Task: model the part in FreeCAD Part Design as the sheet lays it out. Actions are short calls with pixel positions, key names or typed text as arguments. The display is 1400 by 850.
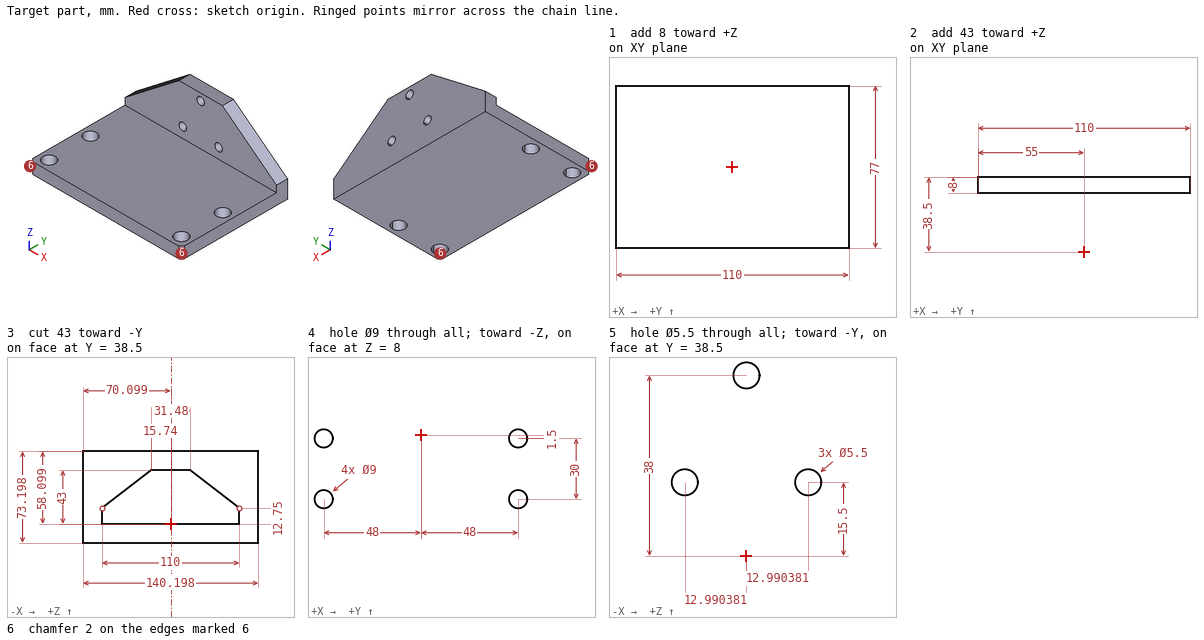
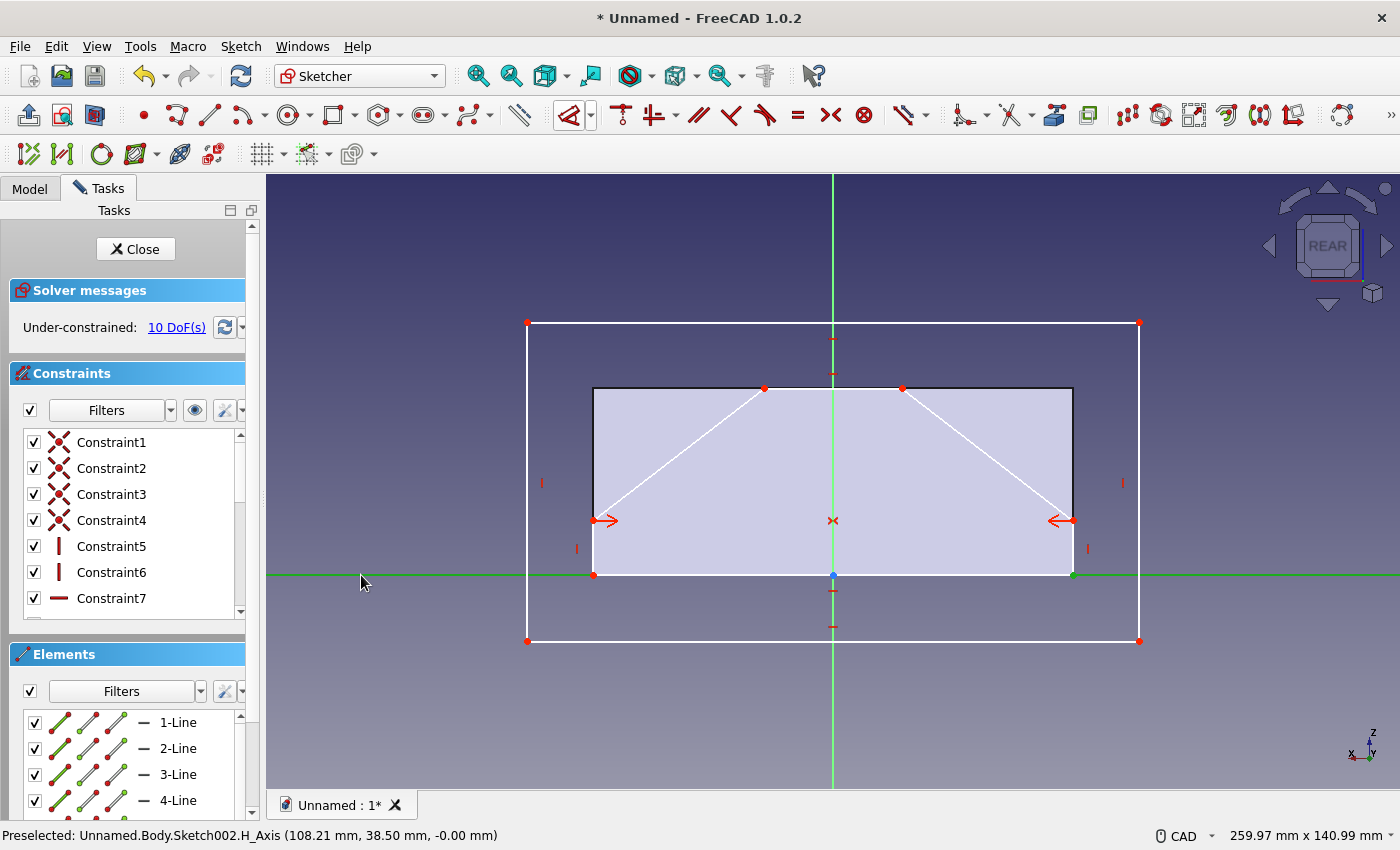
click(621, 116)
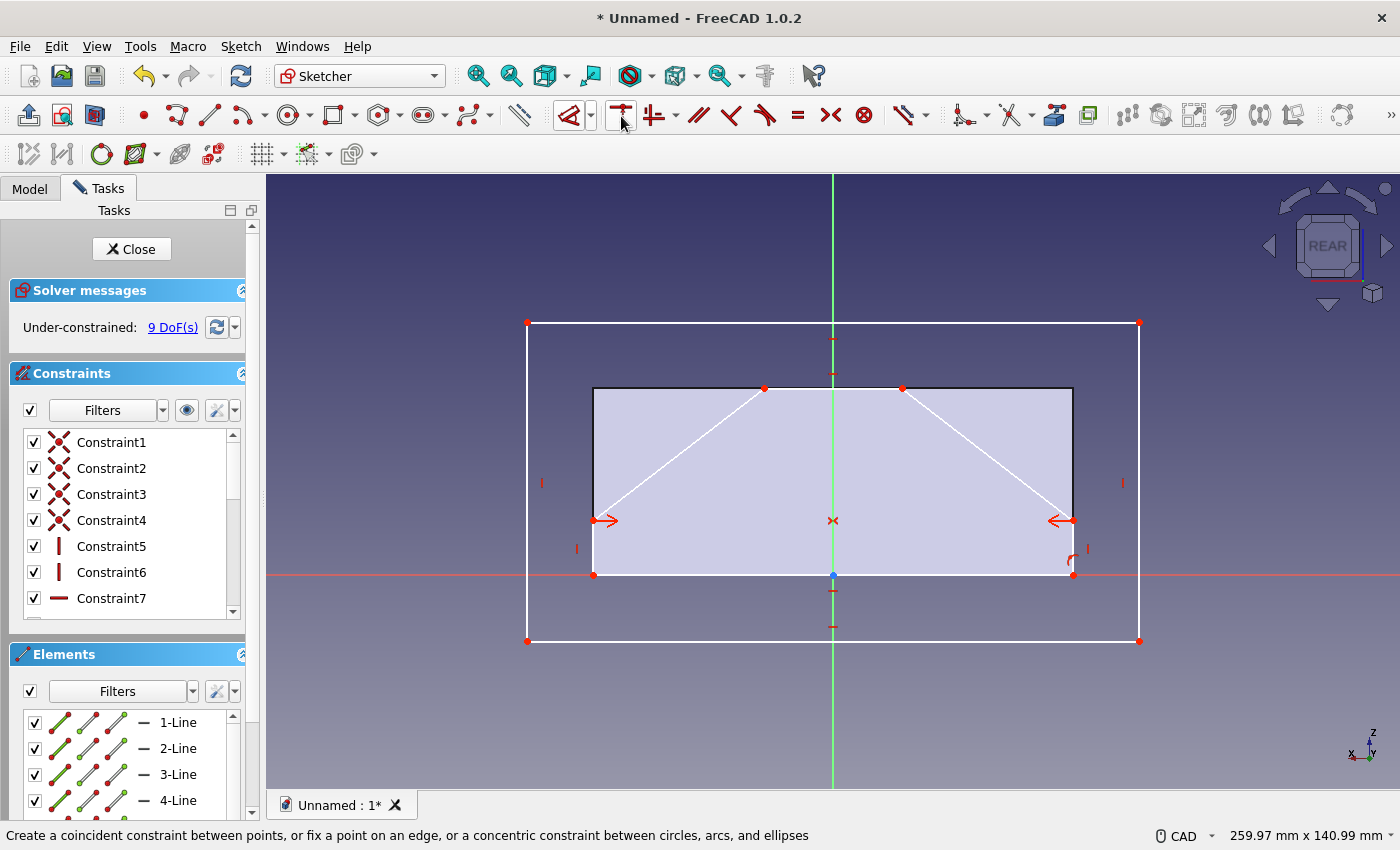
click(929, 575)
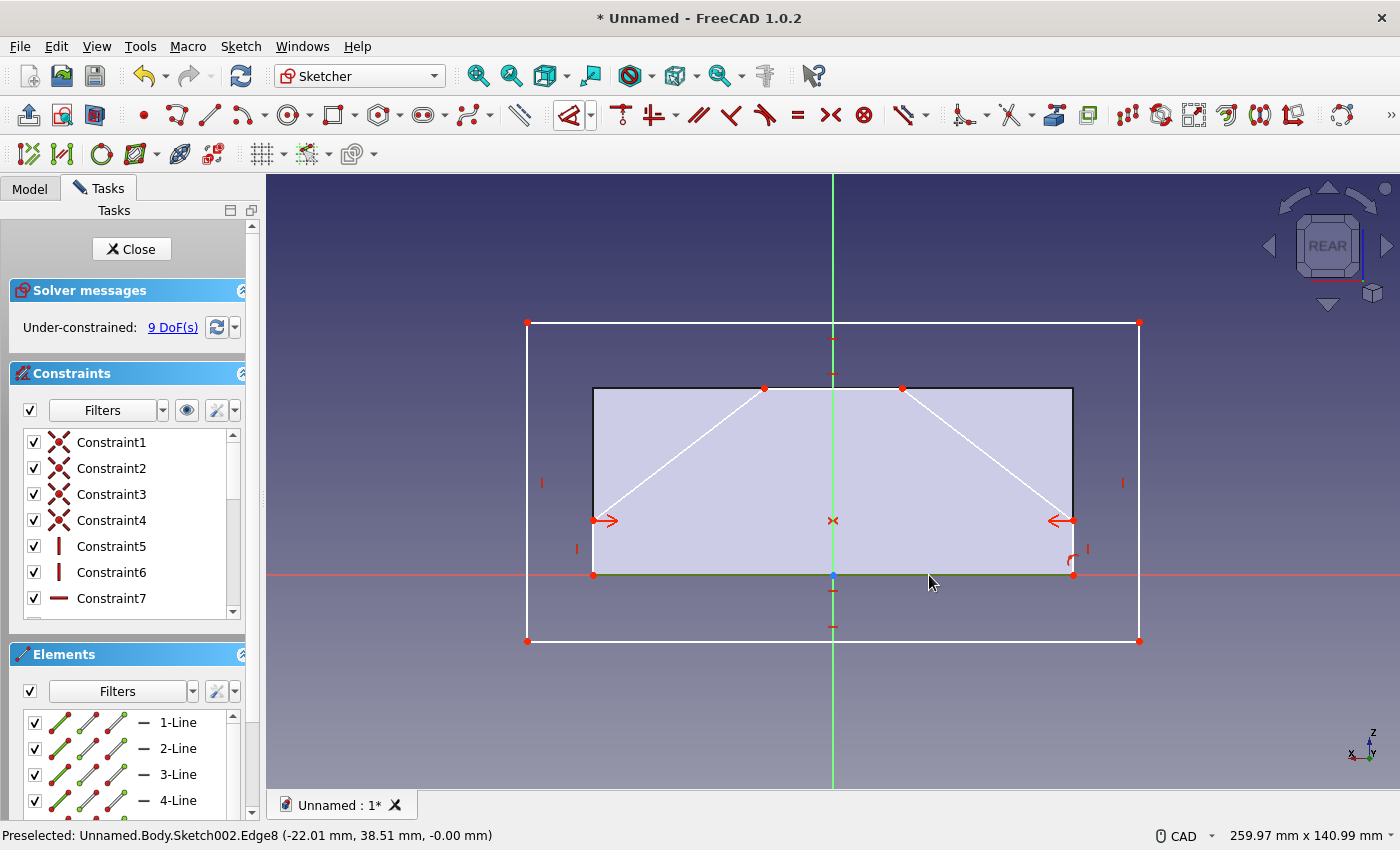
key(l)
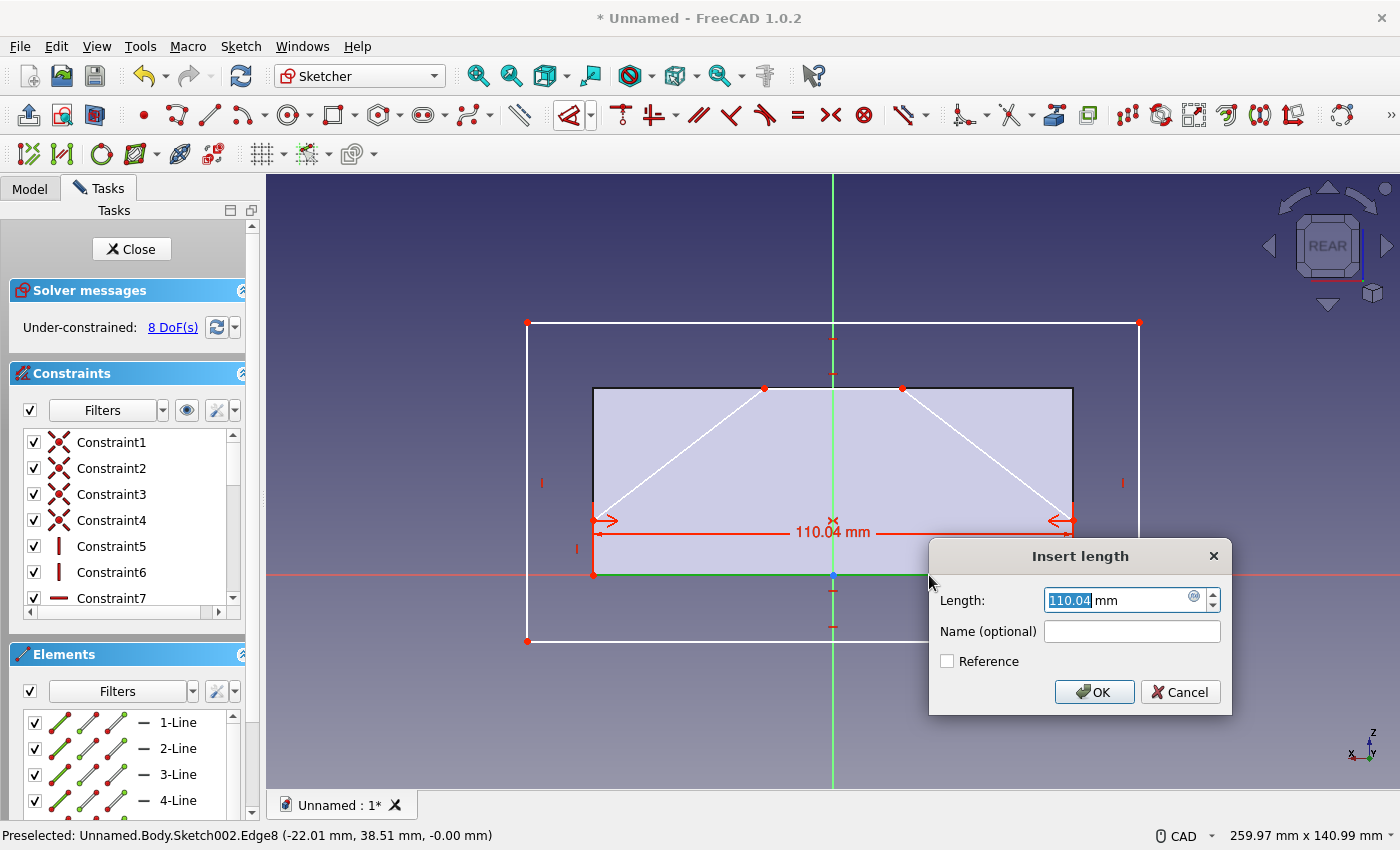
text(110)
key(Return)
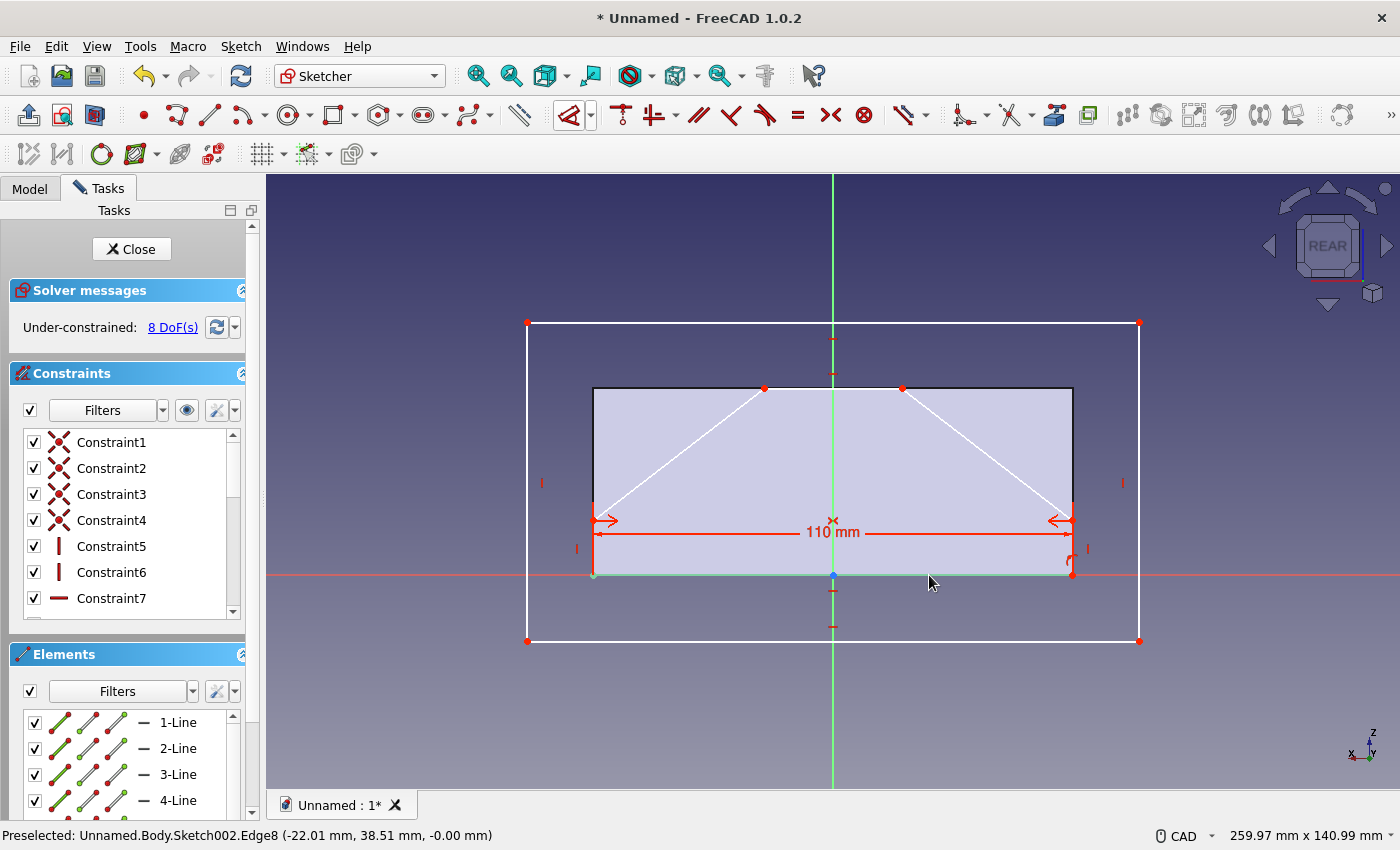
click(764, 389)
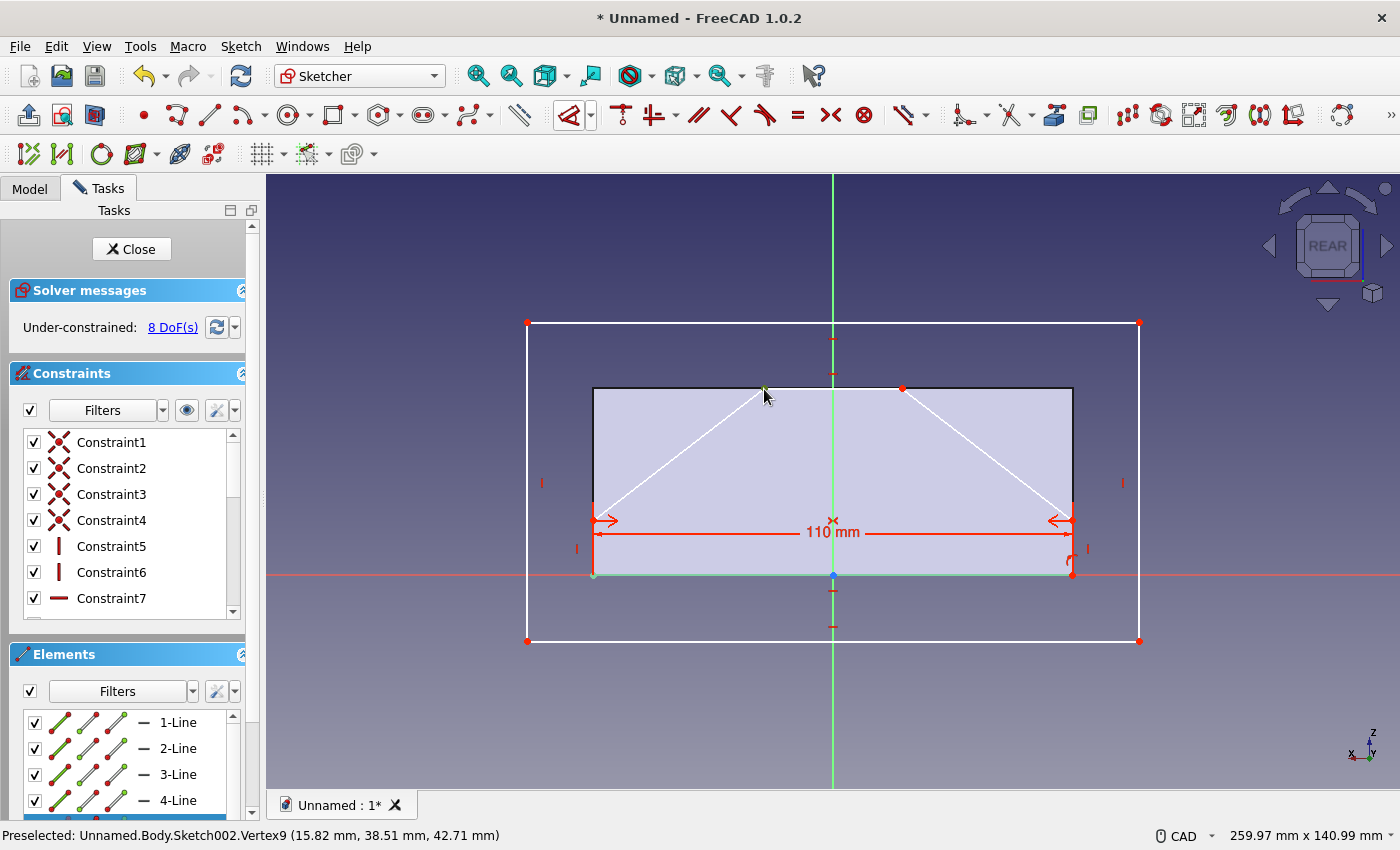
key(i)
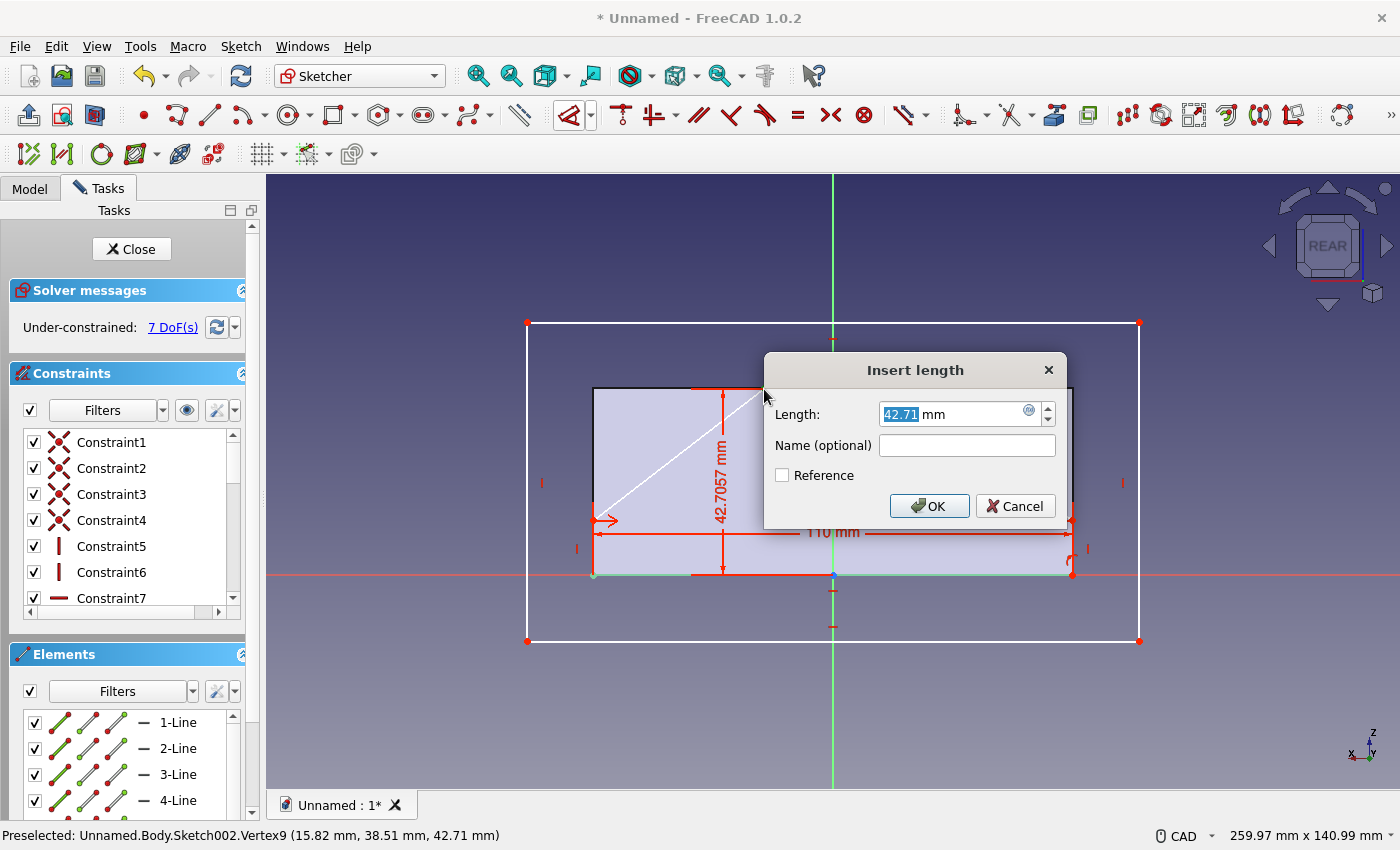
text(43)
key(Return)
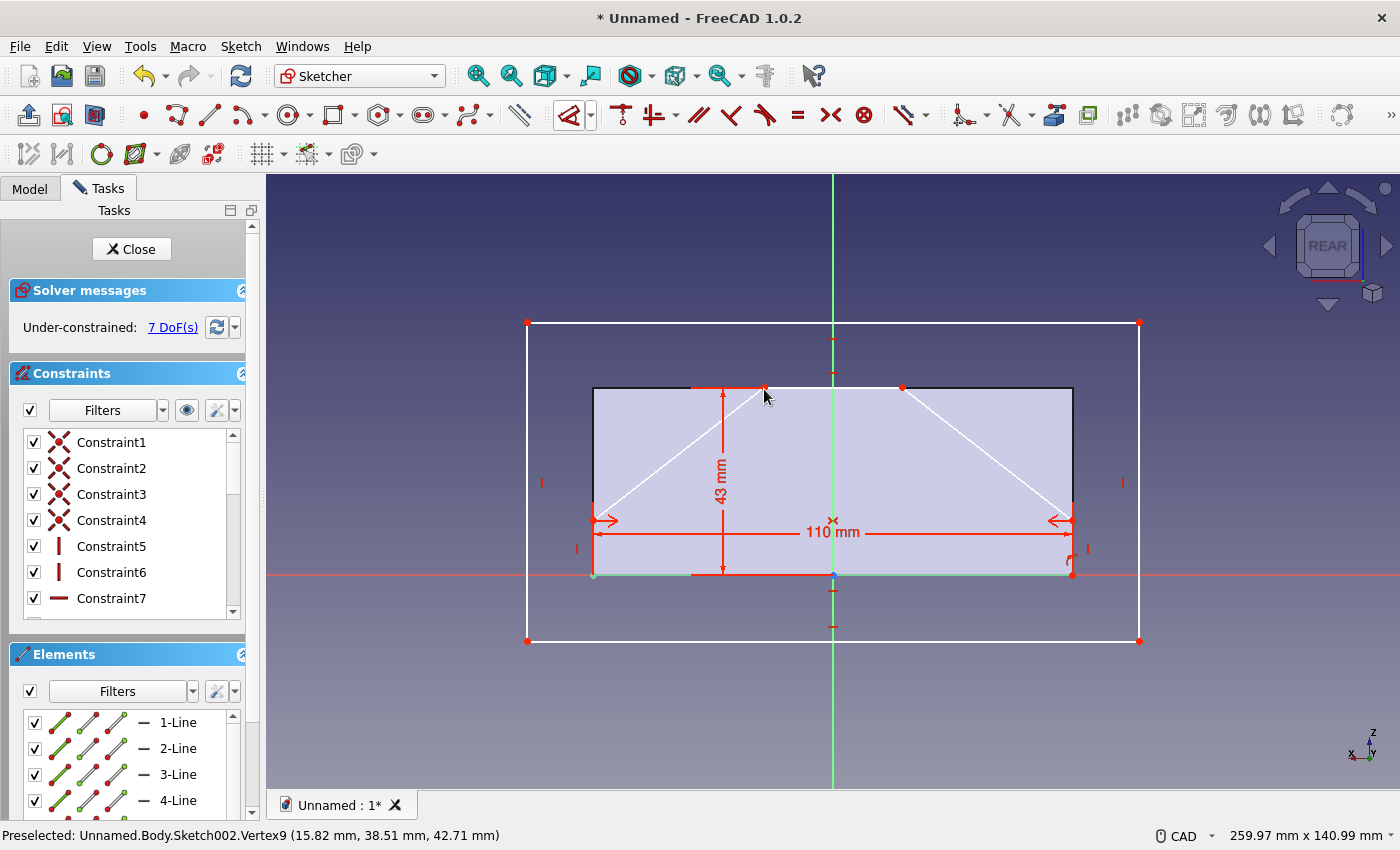
click(805, 388)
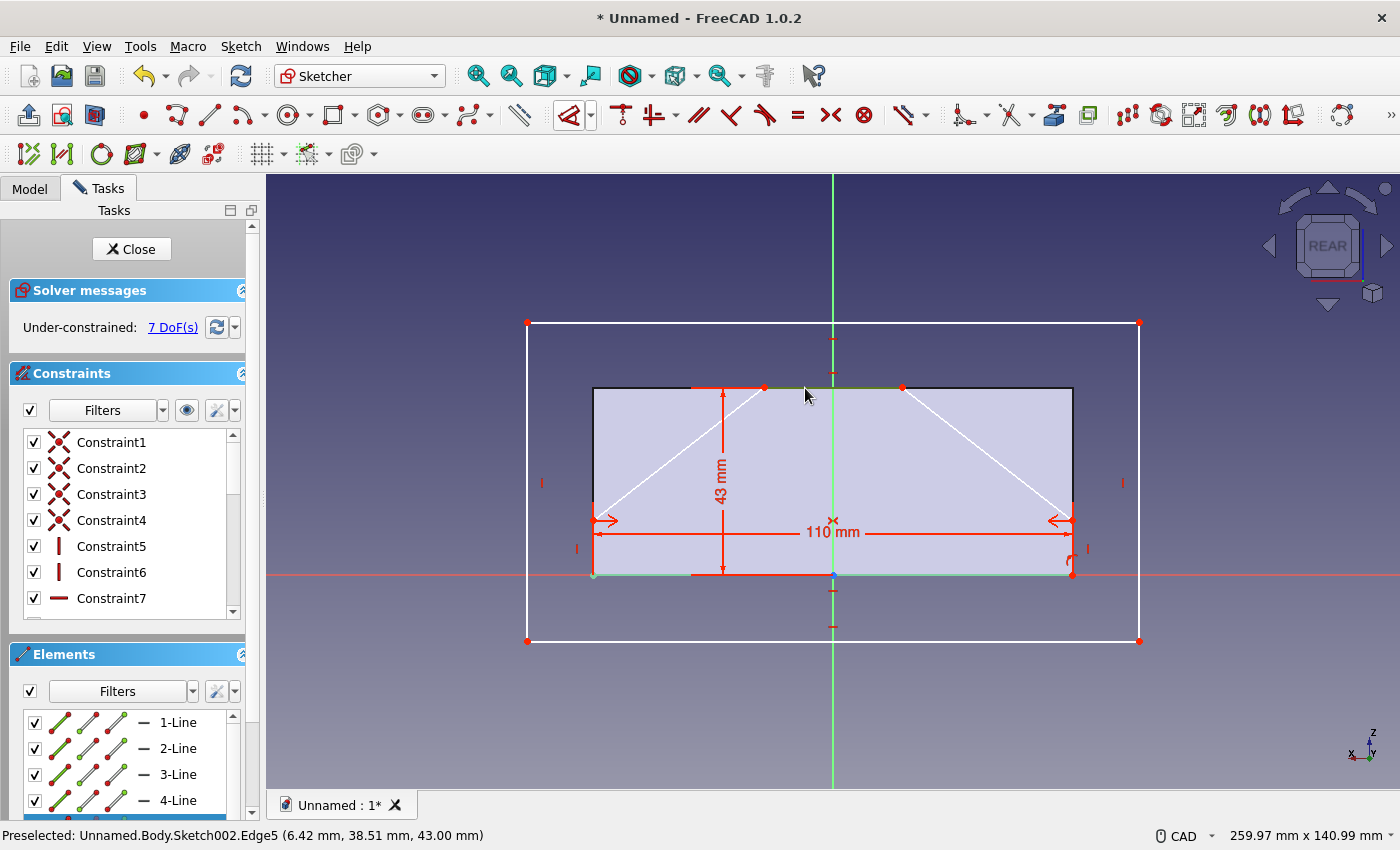
click(590, 116)